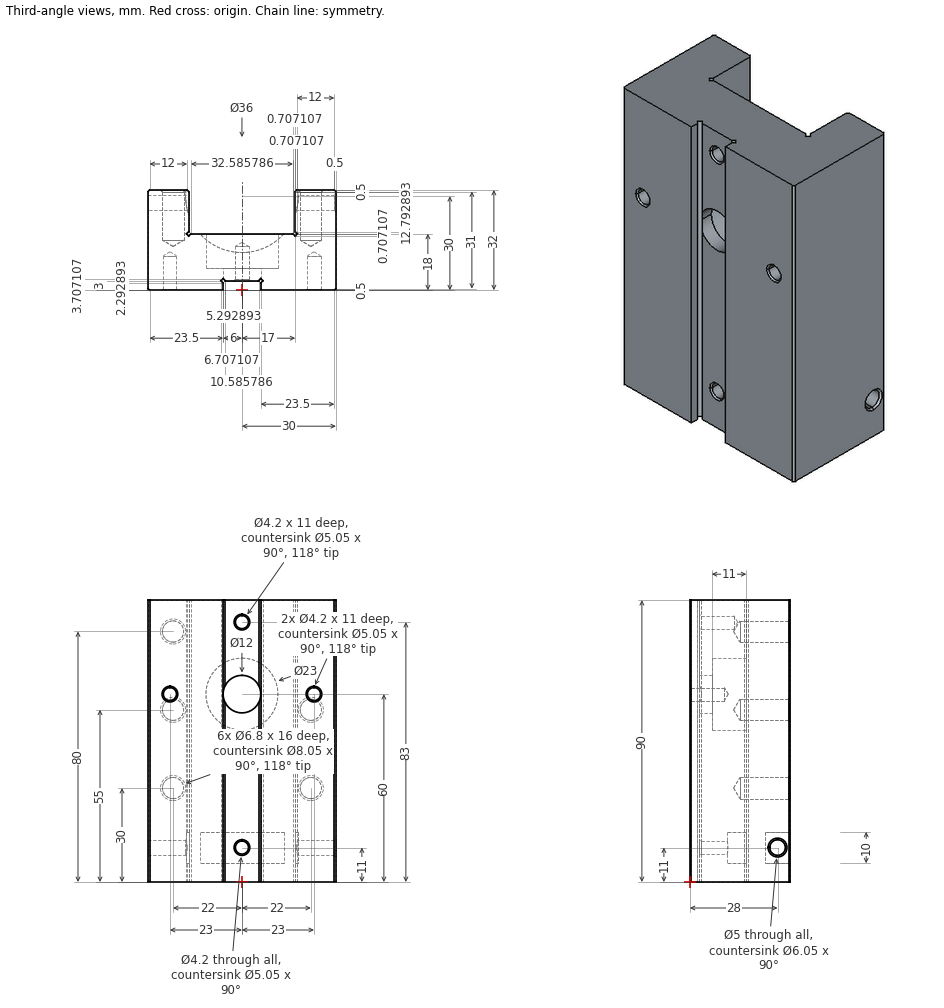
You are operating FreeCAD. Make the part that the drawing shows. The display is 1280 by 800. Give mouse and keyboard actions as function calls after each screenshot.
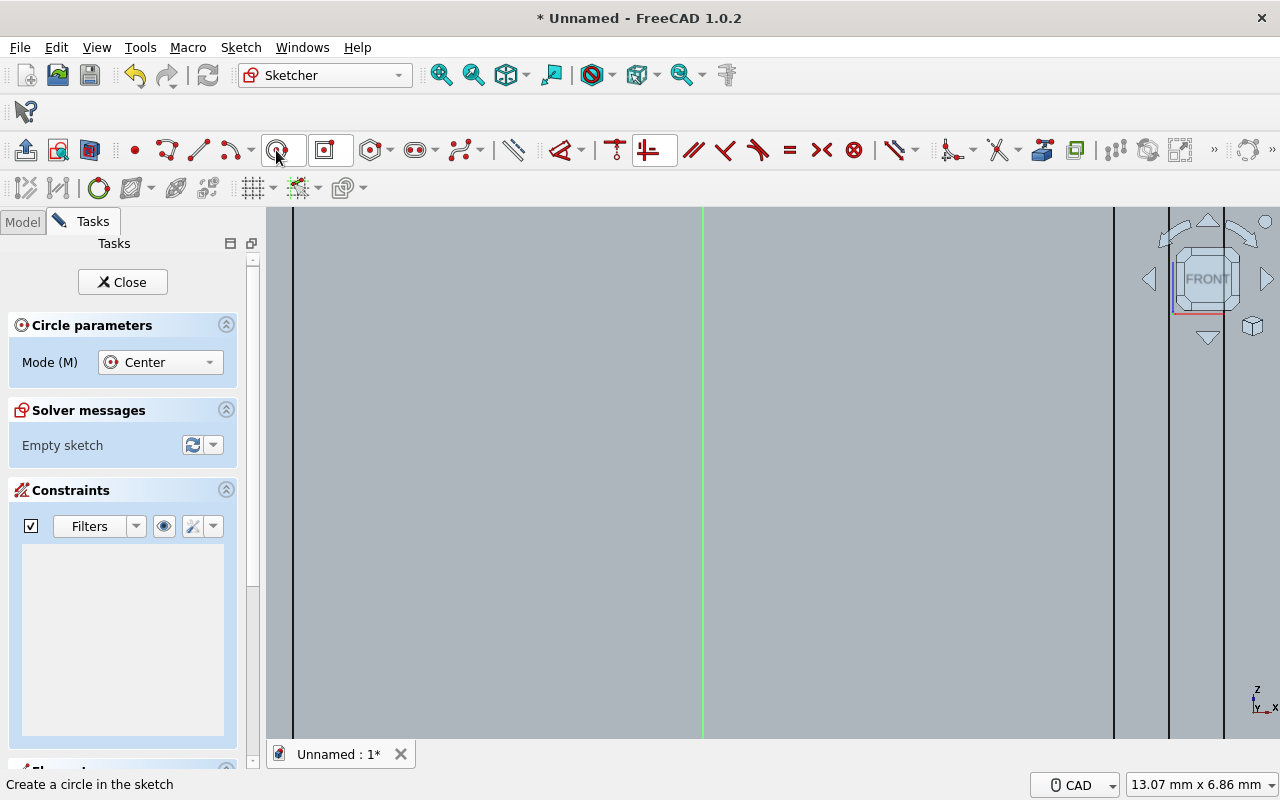
click(703, 474)
move(819, 358)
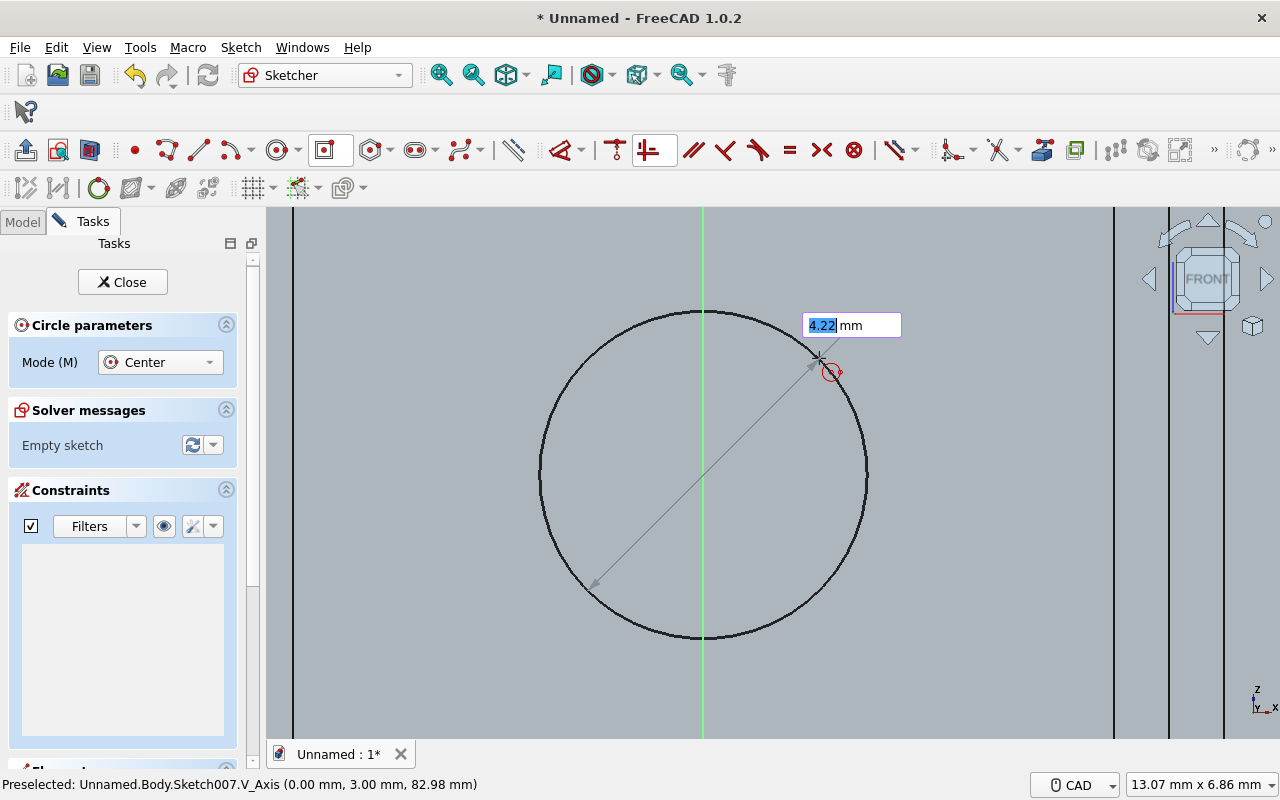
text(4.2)
key(Return)
key(Escape)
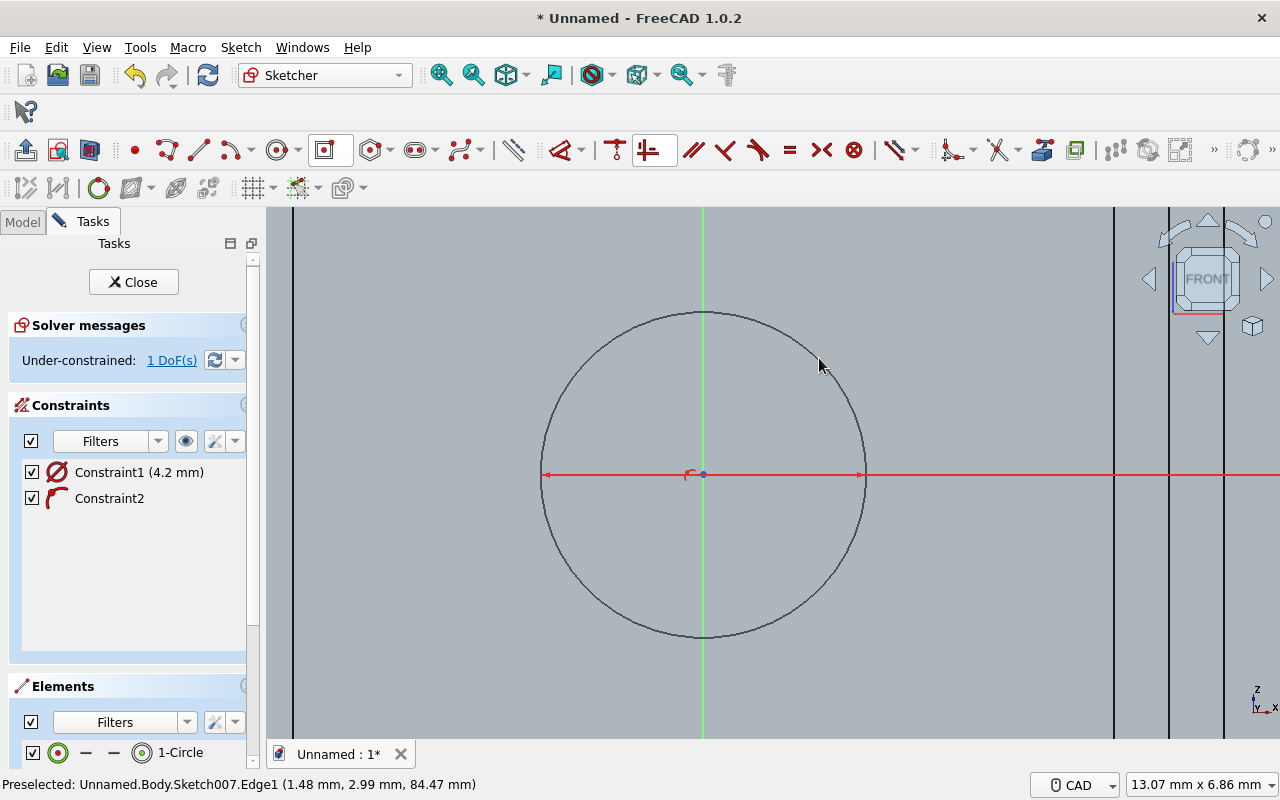
click(560, 150)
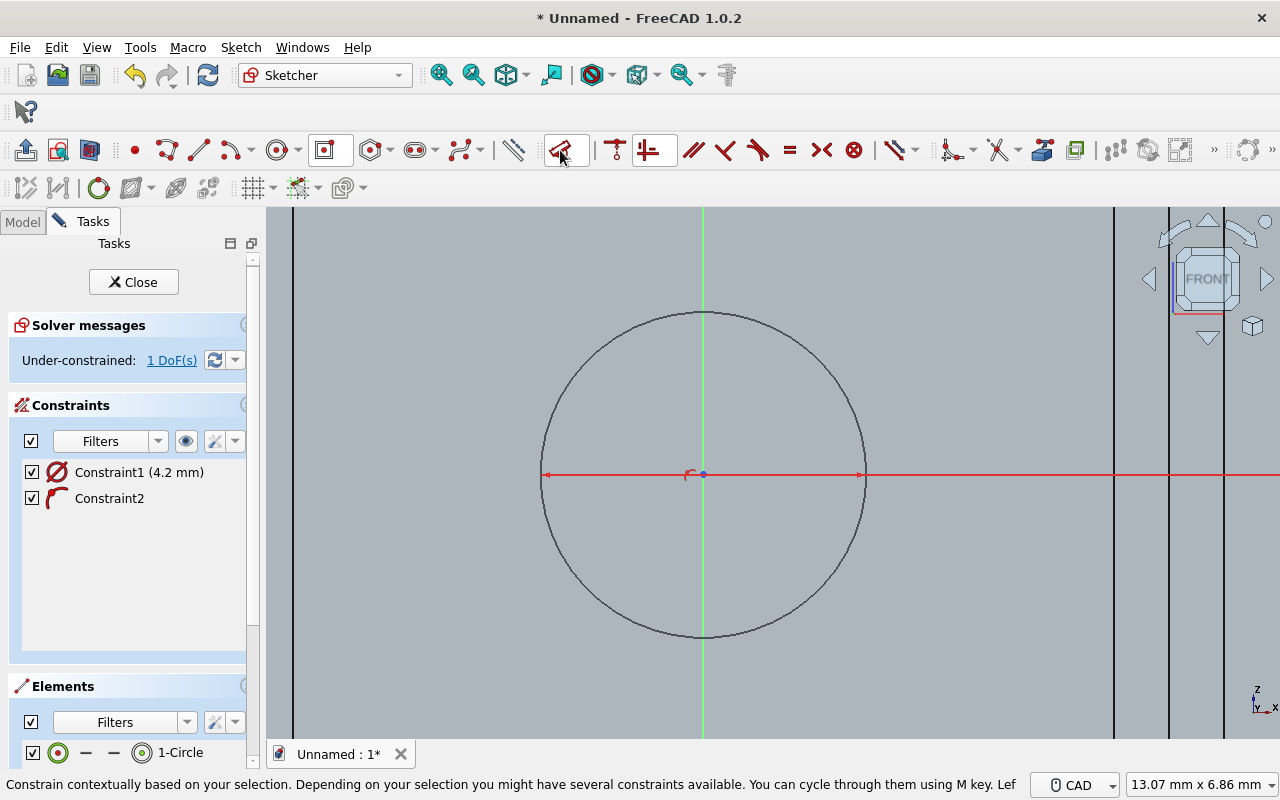
click(703, 475)
click(737, 593)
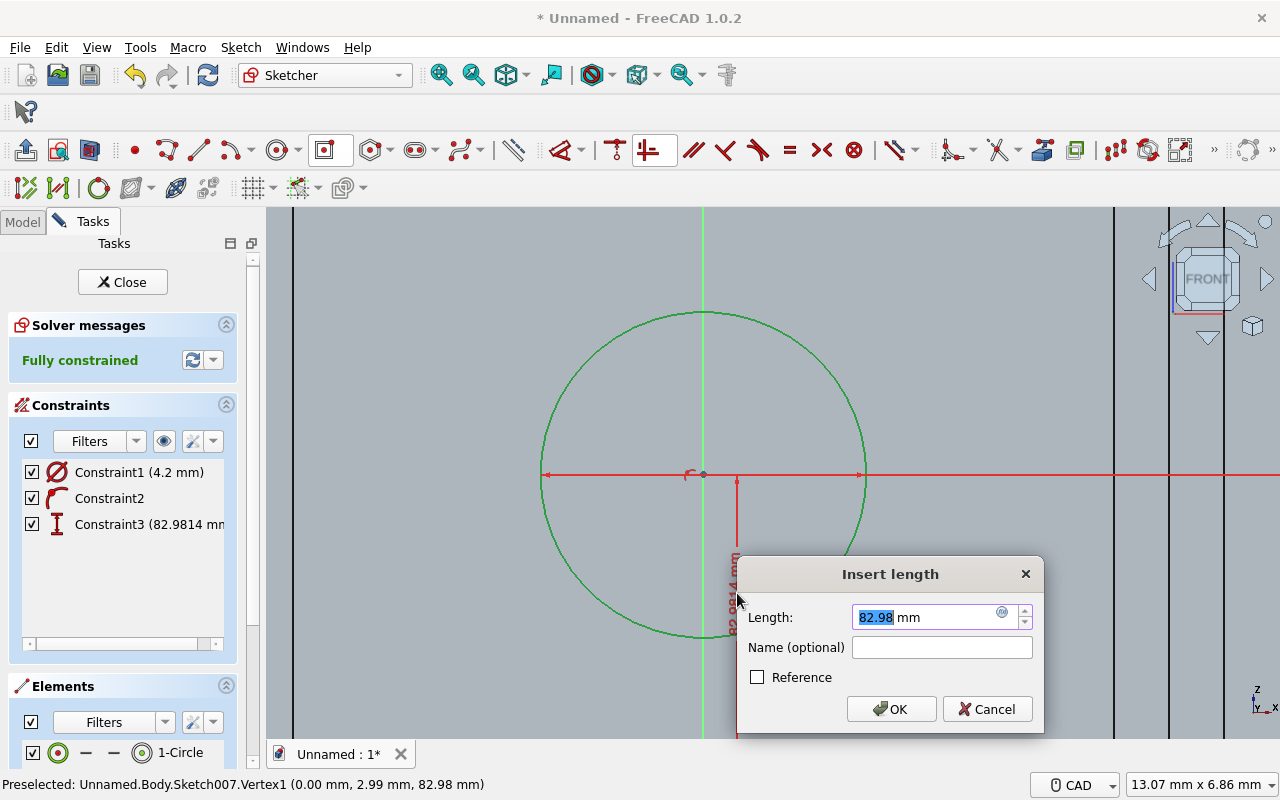
text(83)
key(Return)
key(Escape)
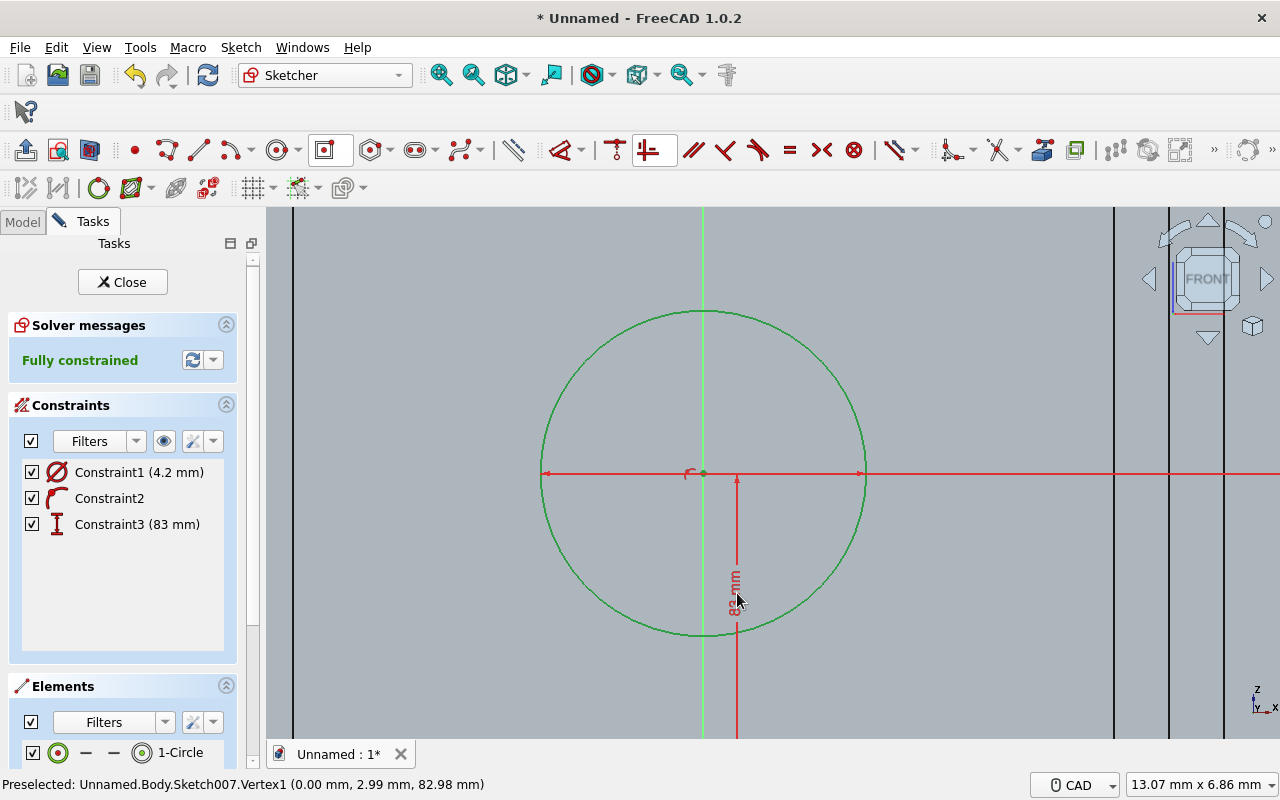
click(123, 282)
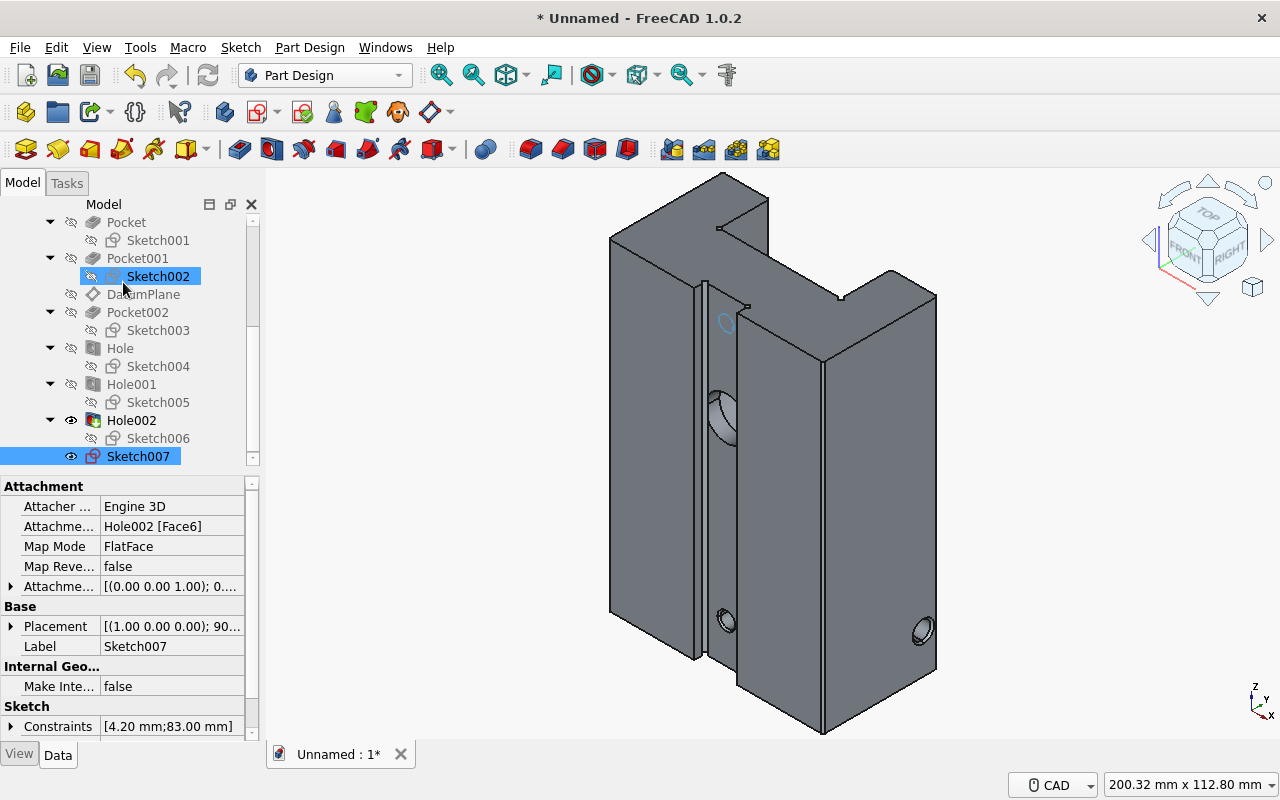
click(272, 150)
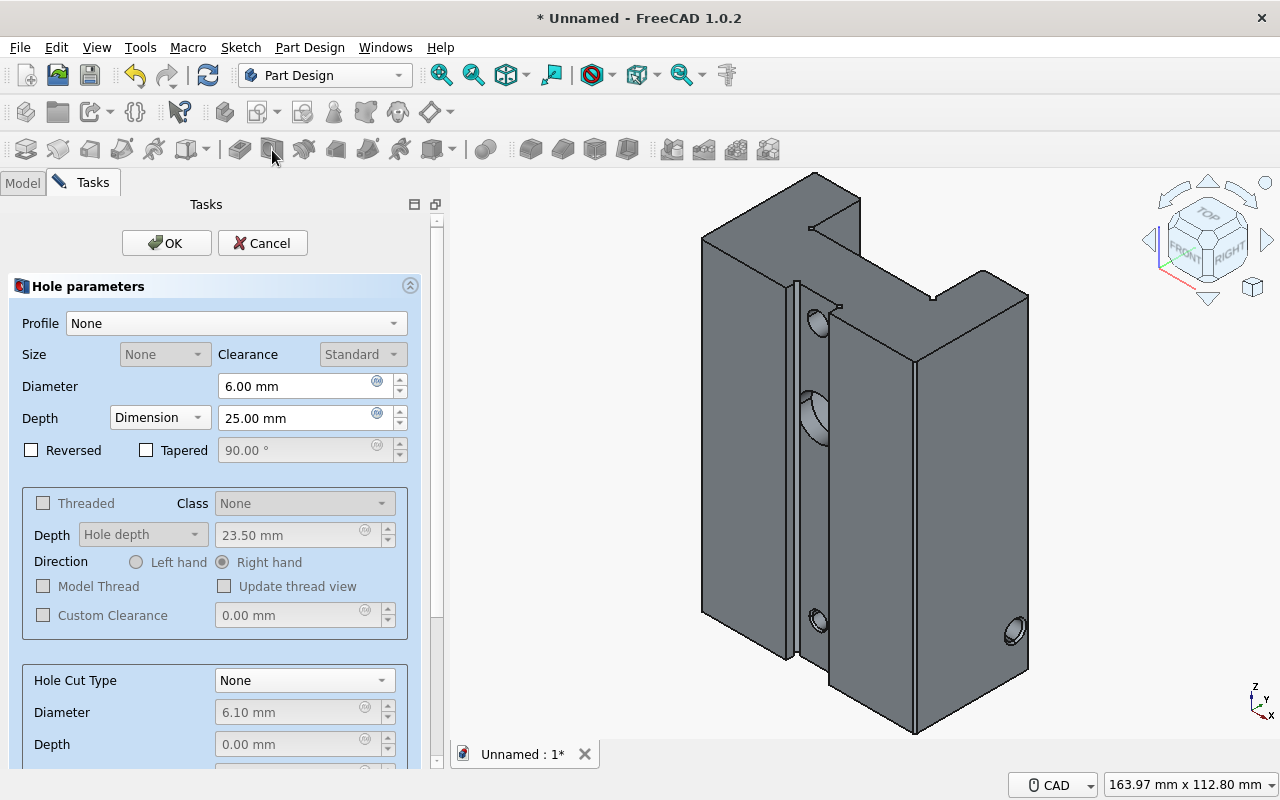
triple_click(305, 386)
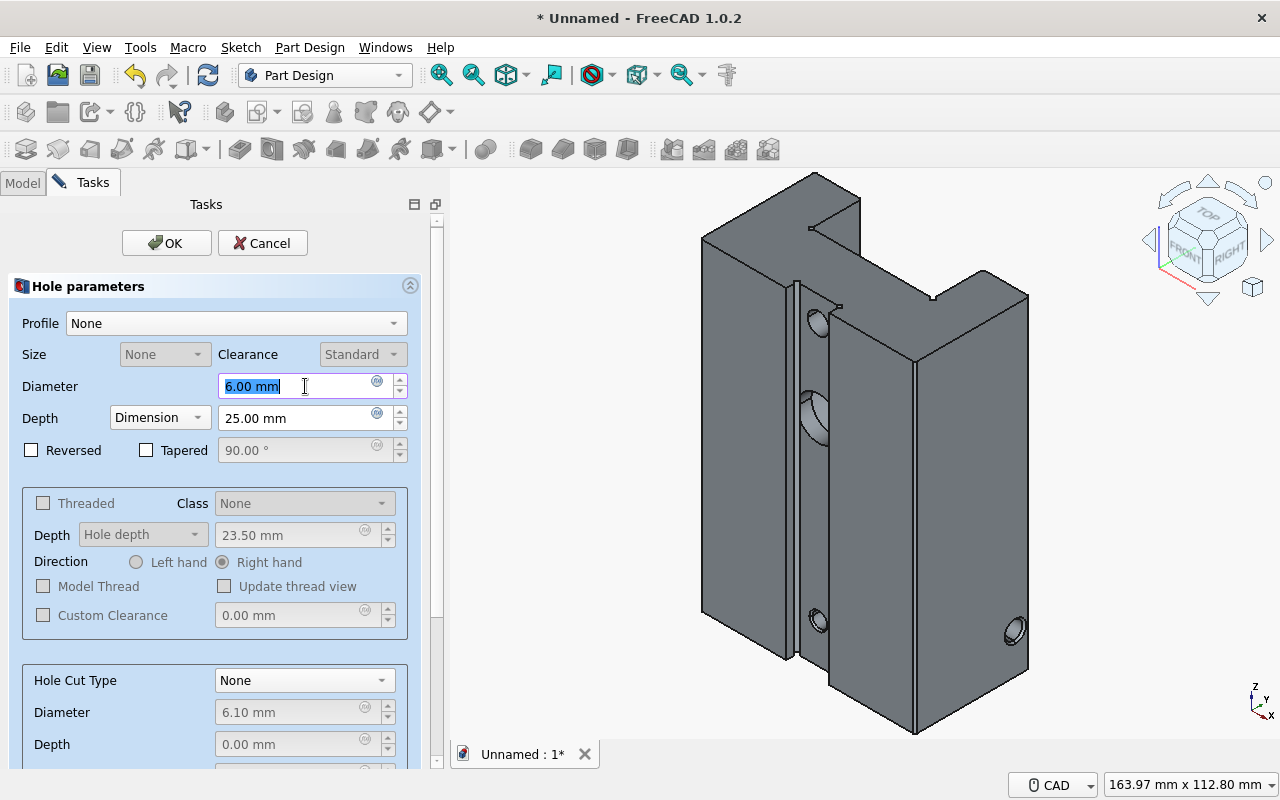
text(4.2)
key(Tab)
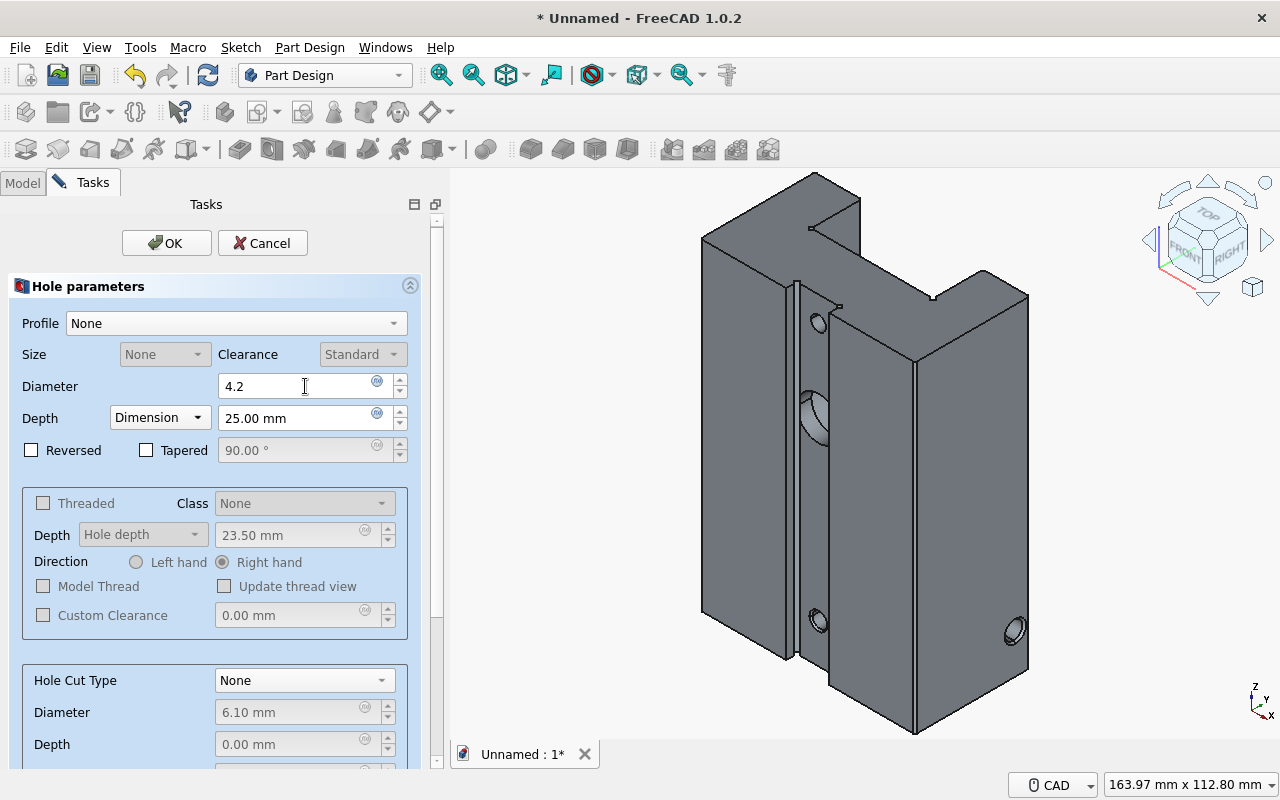
triple_click(305, 418)